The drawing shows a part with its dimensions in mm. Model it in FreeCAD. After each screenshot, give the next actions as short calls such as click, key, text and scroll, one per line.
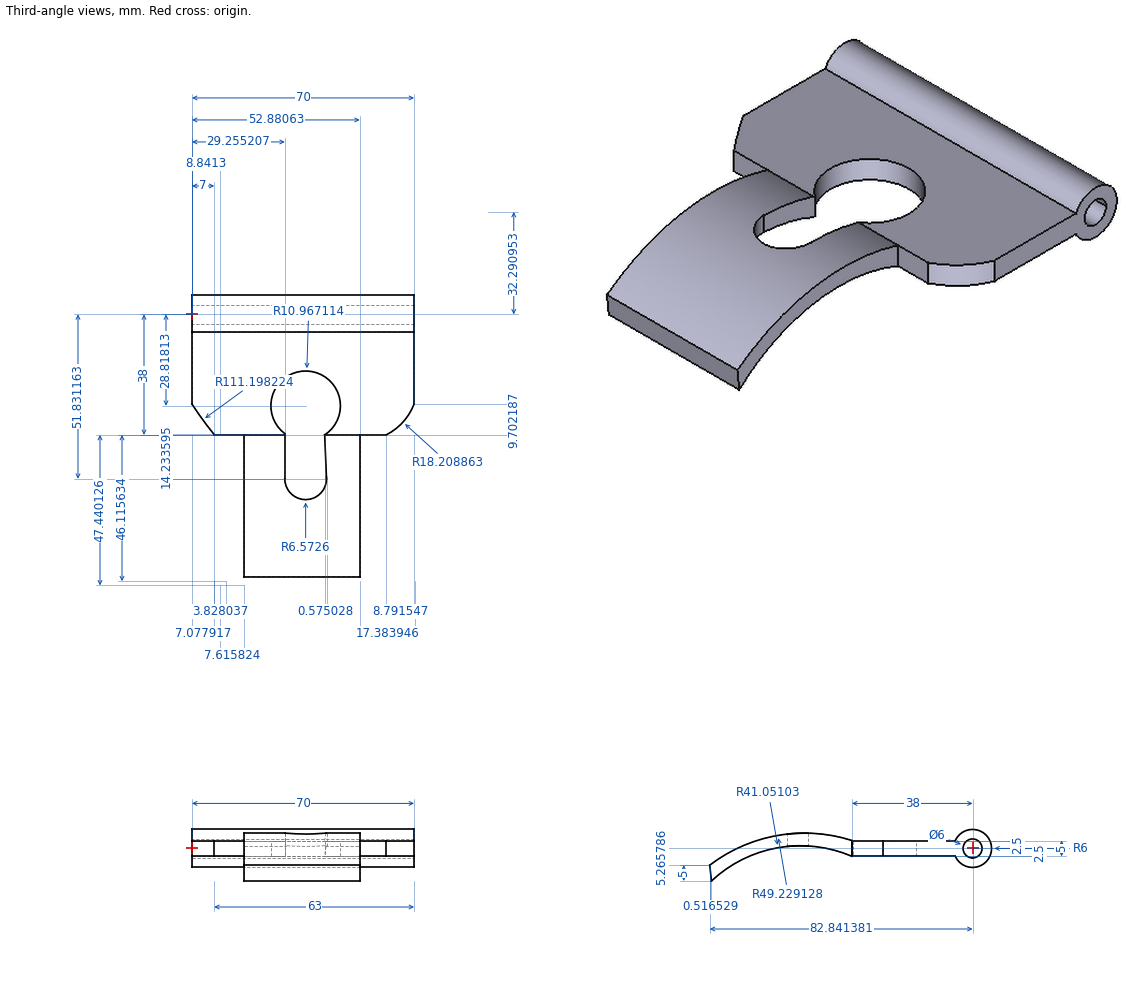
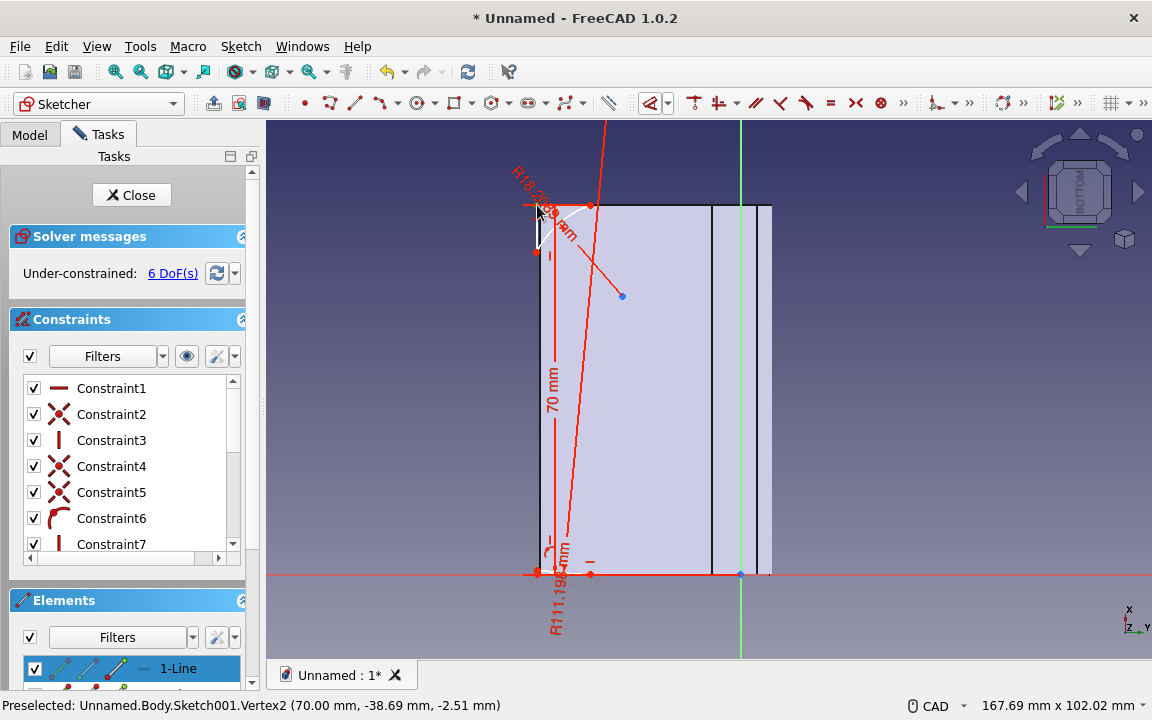
key(l)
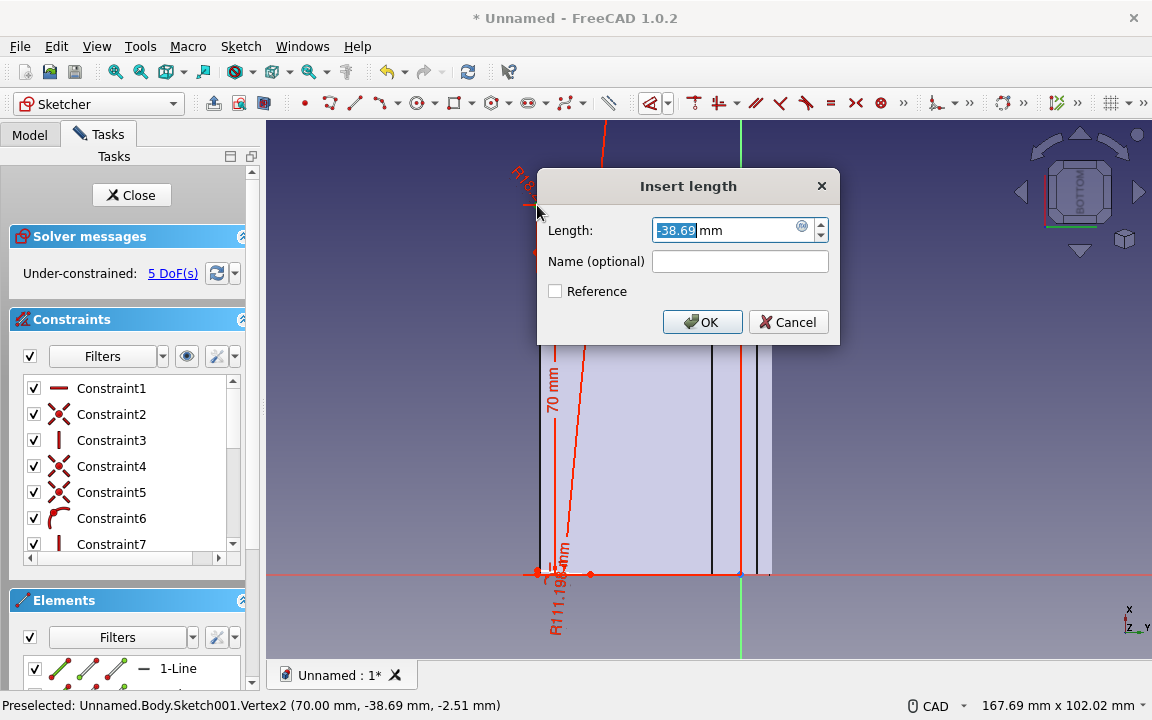
text(-38)
key(Return)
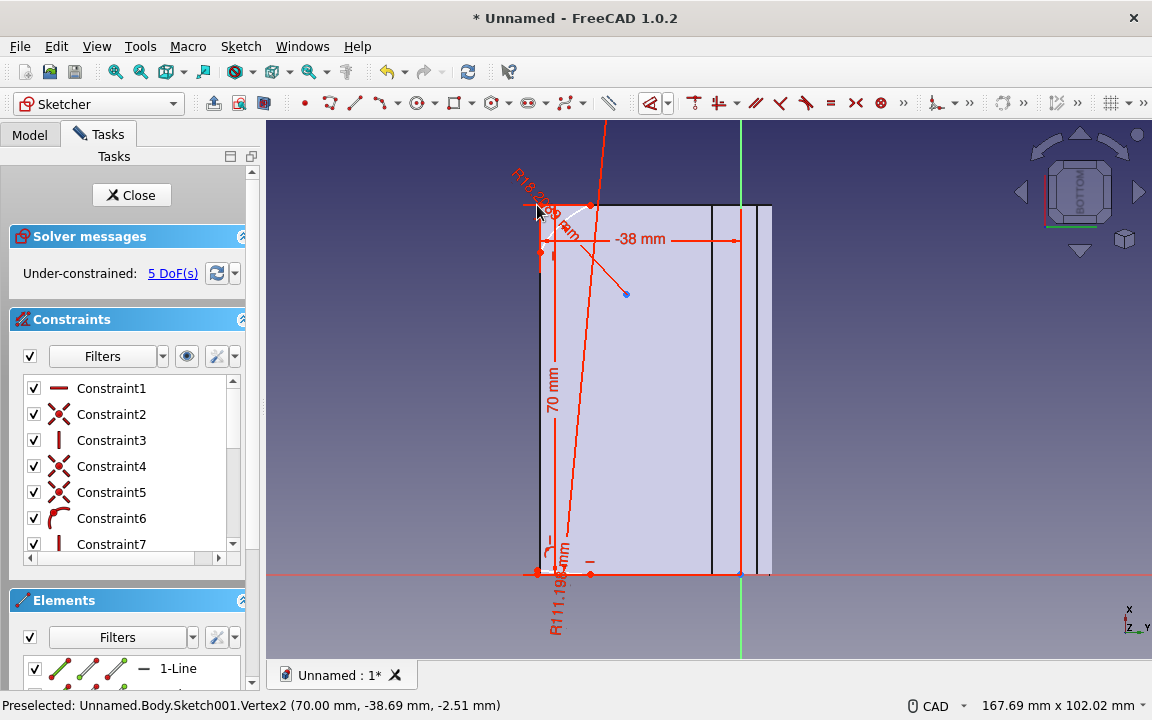
scroll(537, 570, up, 5)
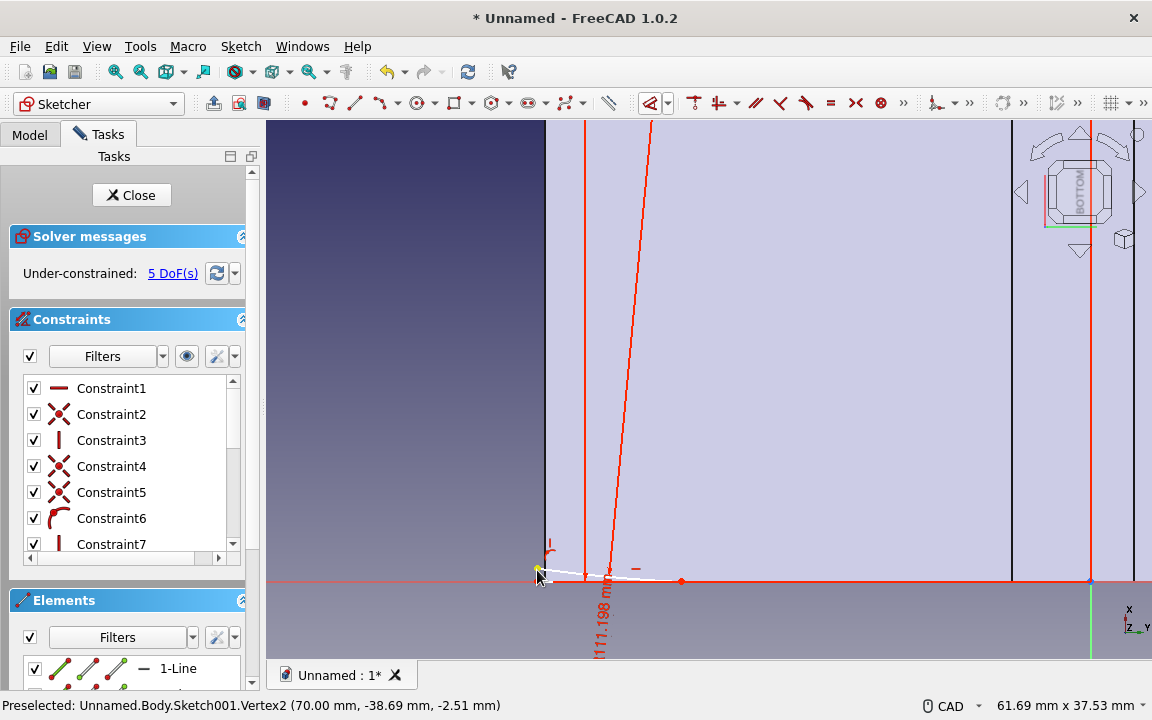
click(537, 569)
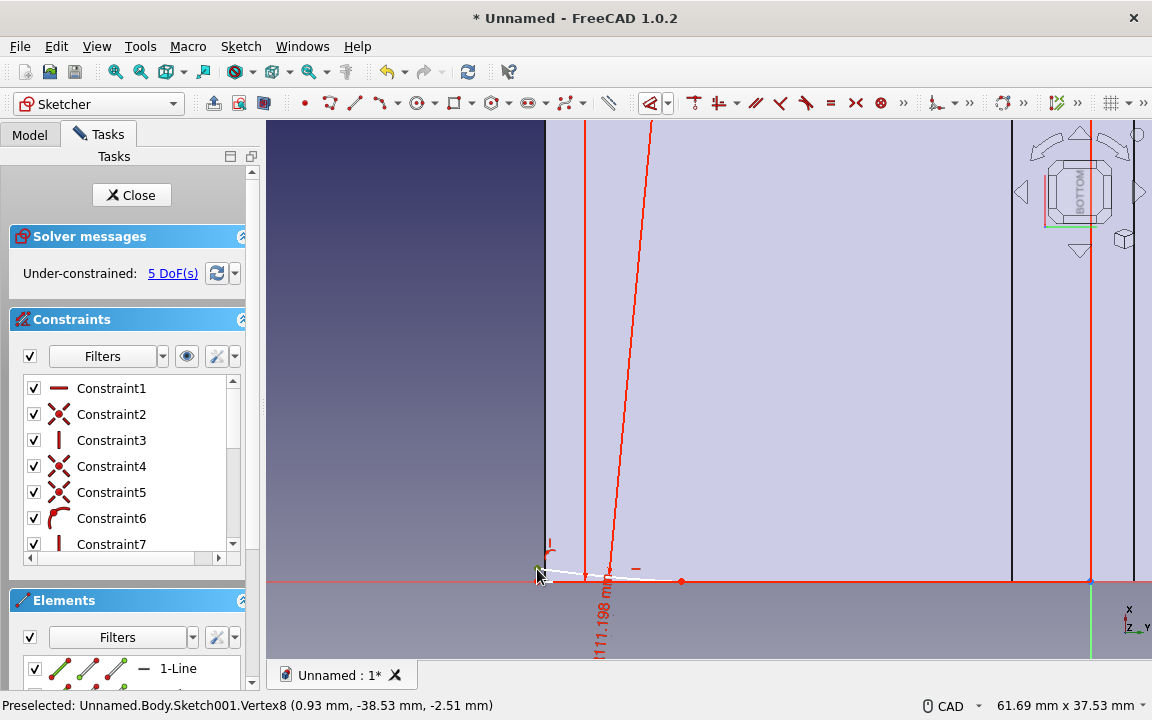
key(l)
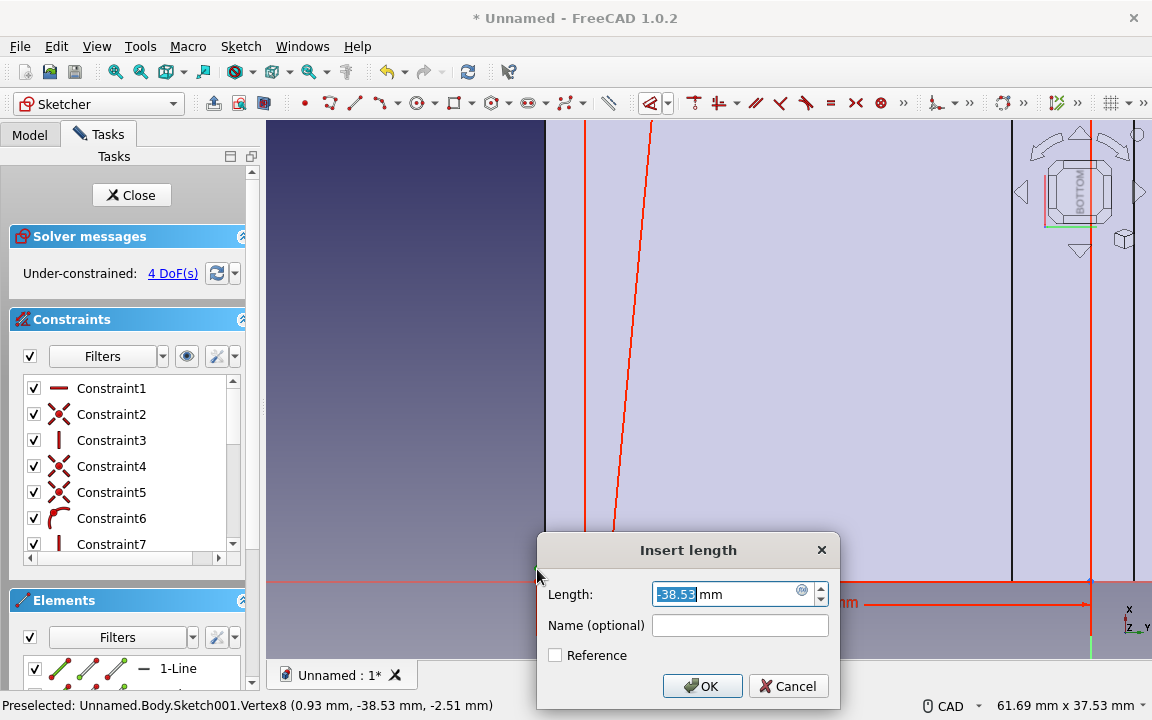
text(-38)
key(Return)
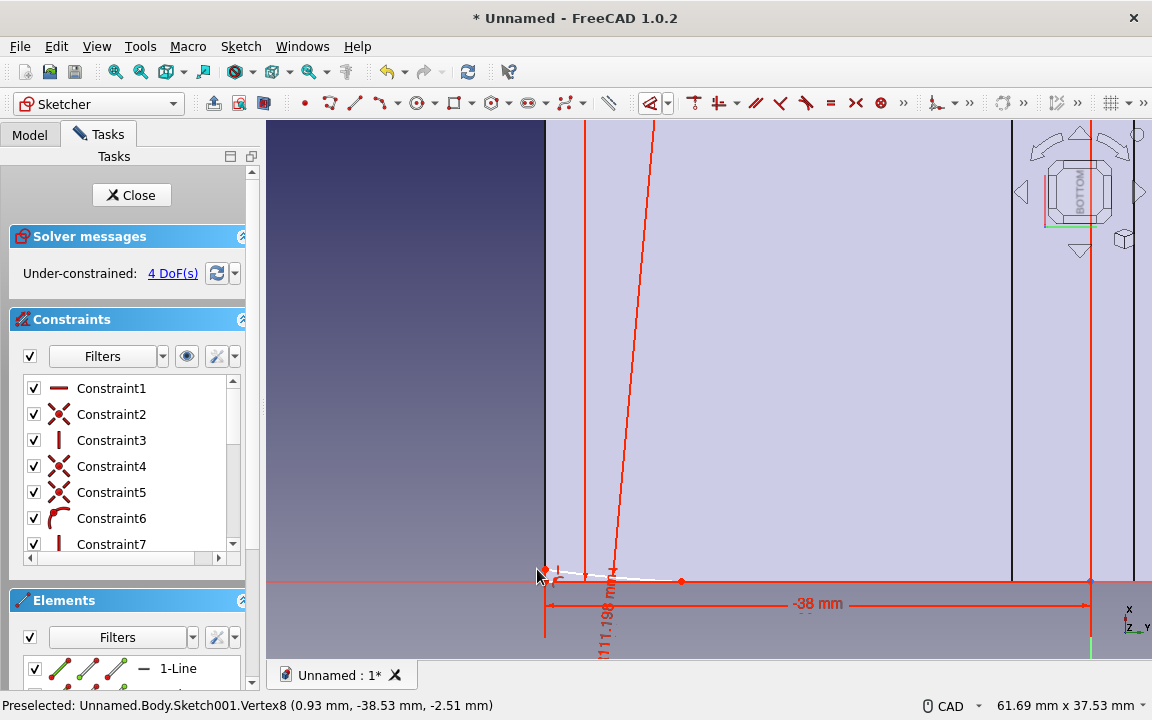
scroll(537, 570, down, 5)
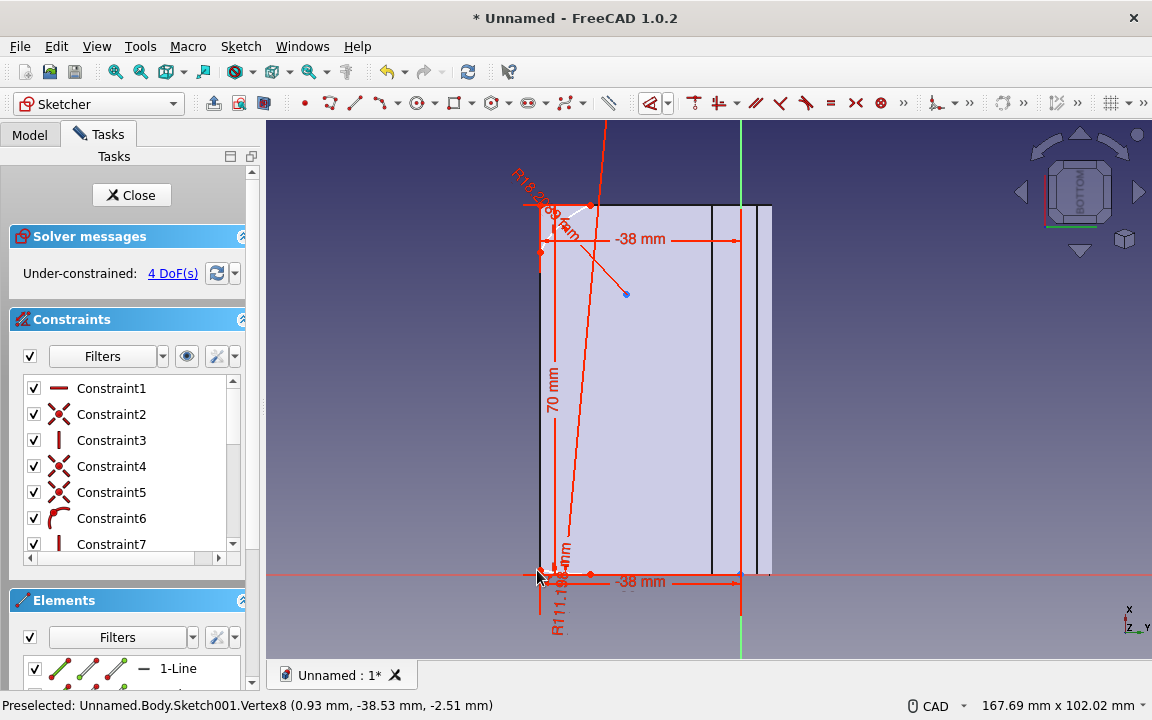
scroll(576, 205, up, 4)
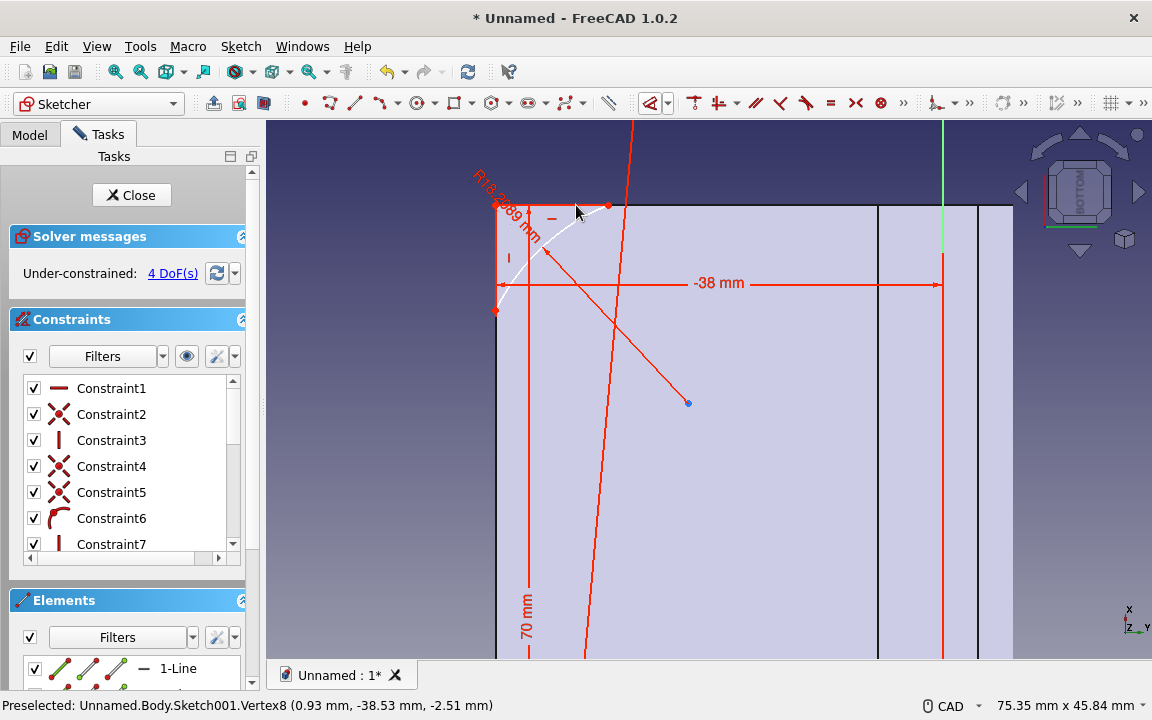
click(575, 205)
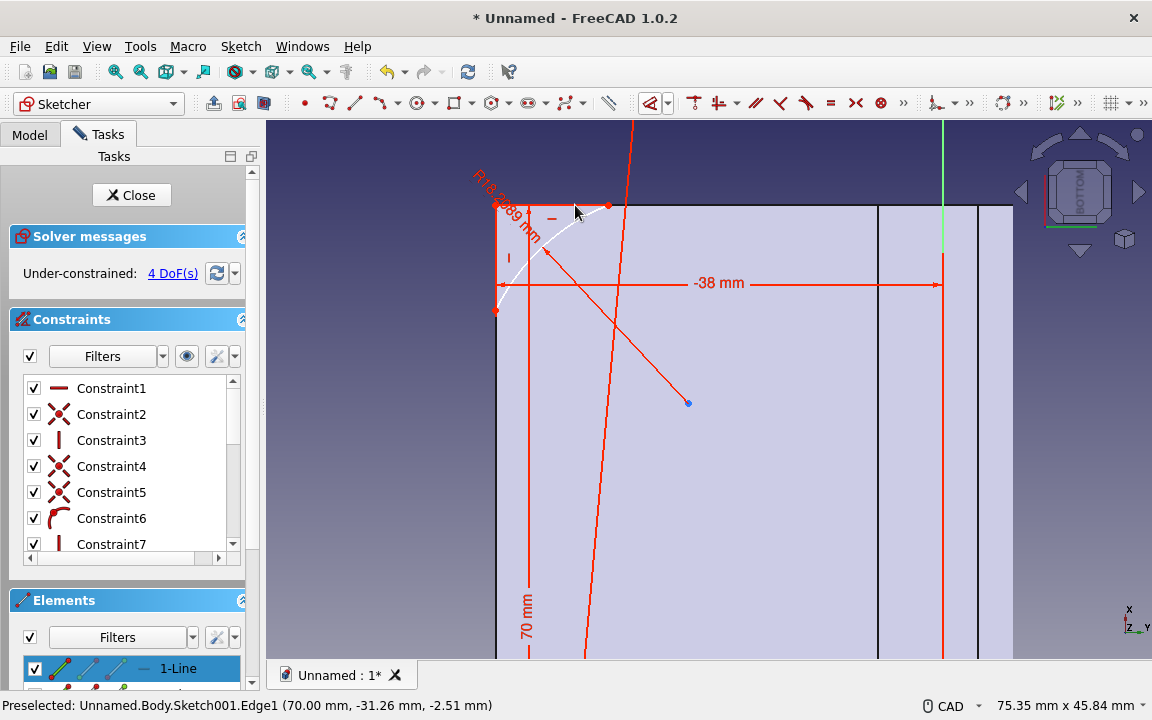
key(l)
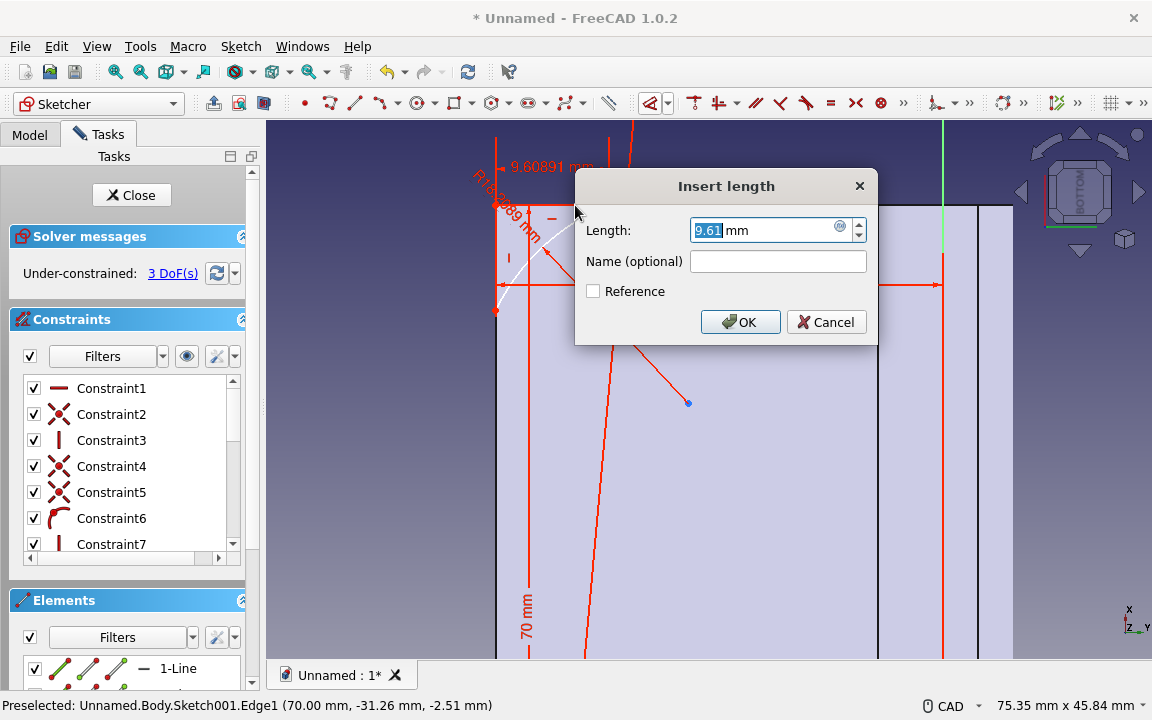
text(9.702187)
key(Return)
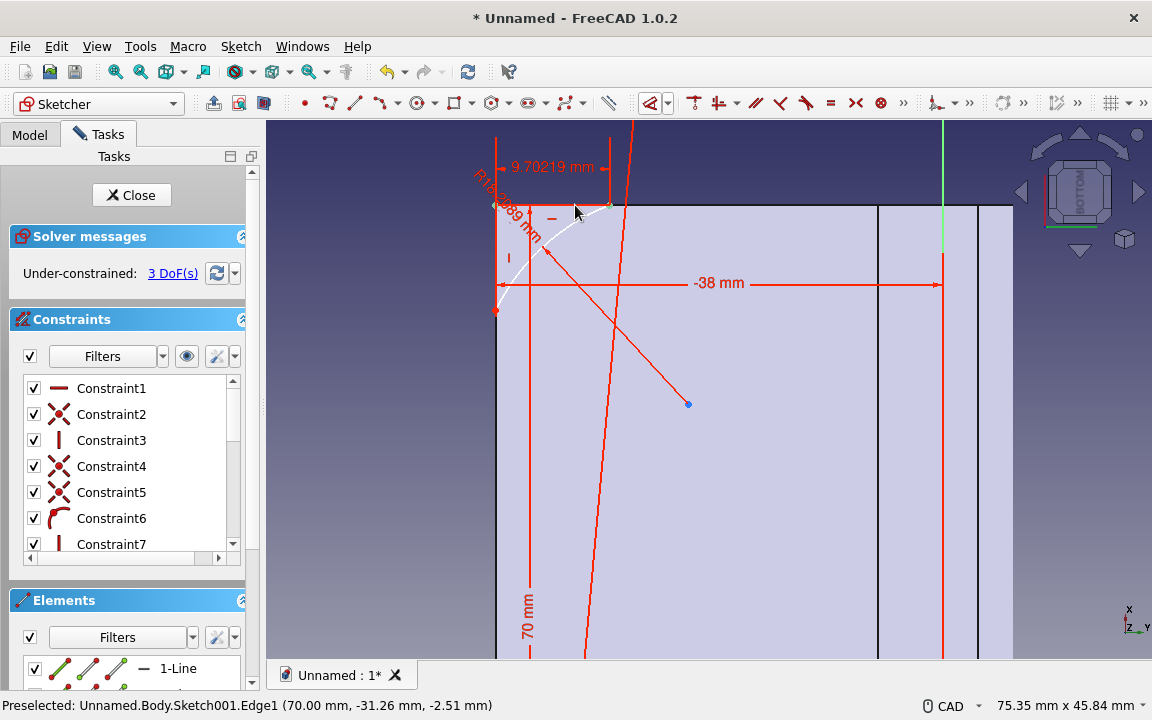
click(496, 237)